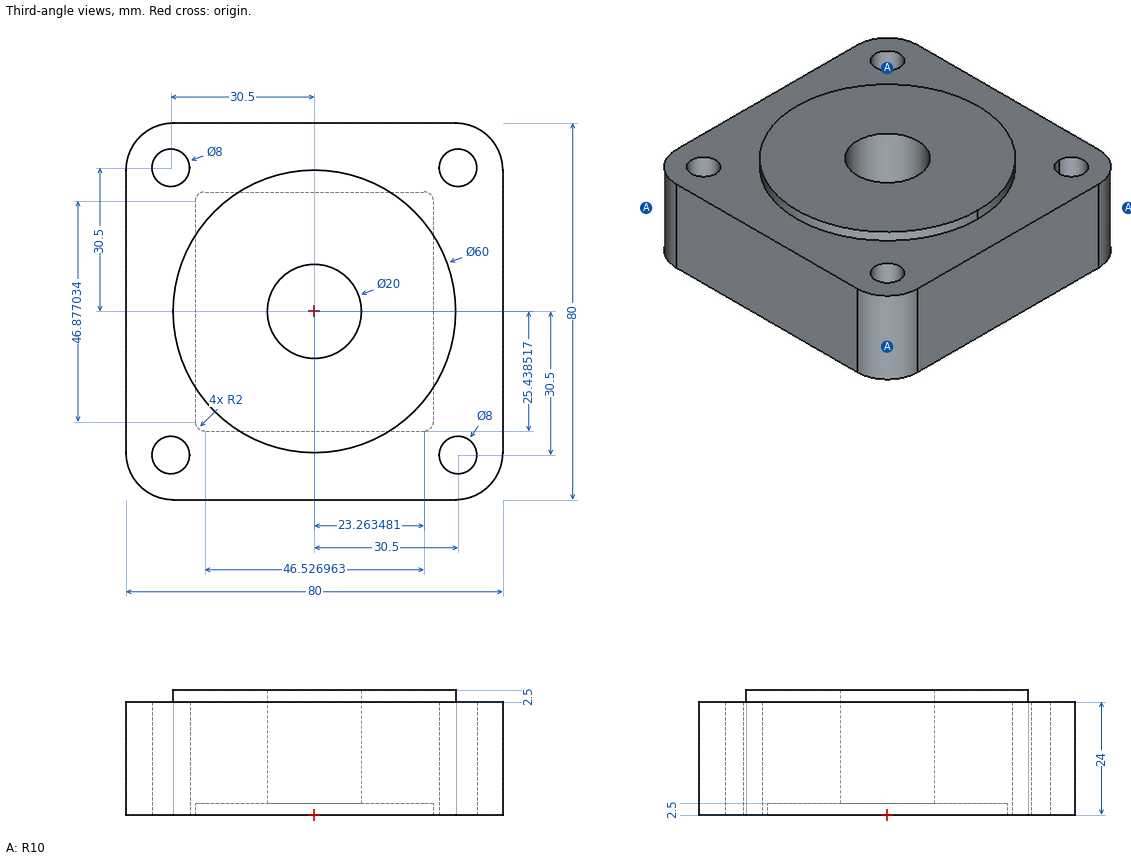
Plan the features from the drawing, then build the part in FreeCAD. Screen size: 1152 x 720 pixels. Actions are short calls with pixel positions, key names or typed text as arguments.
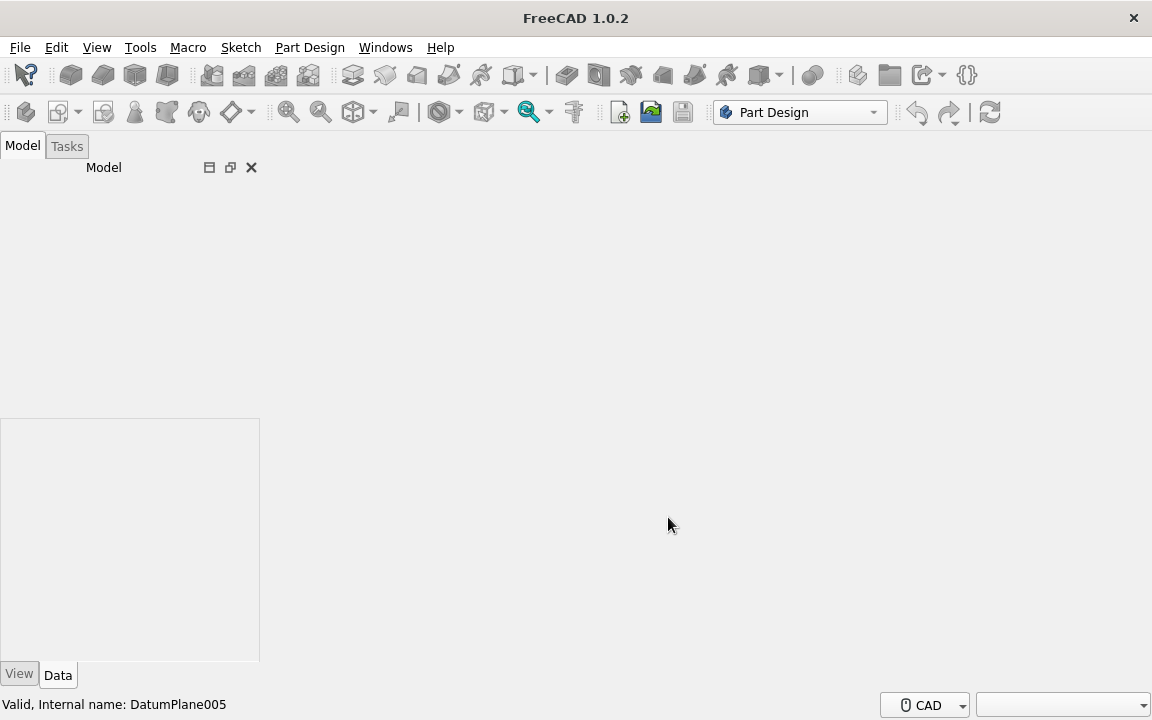
click(620, 112)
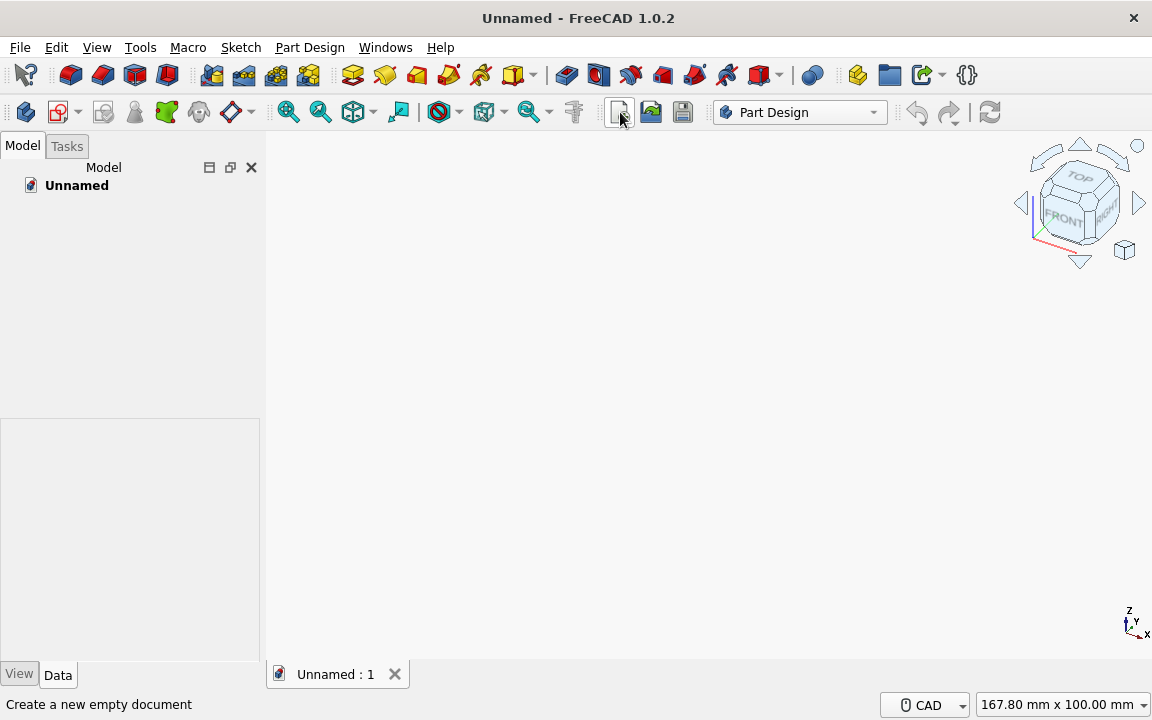
click(58, 112)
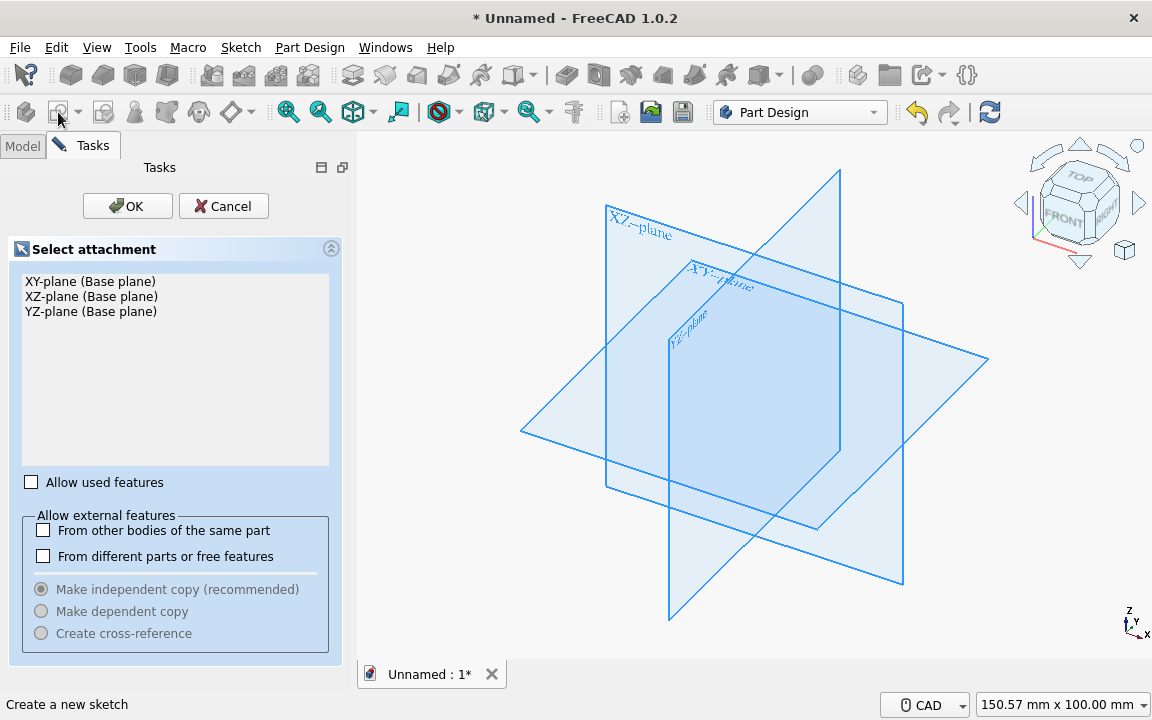
click(82, 282)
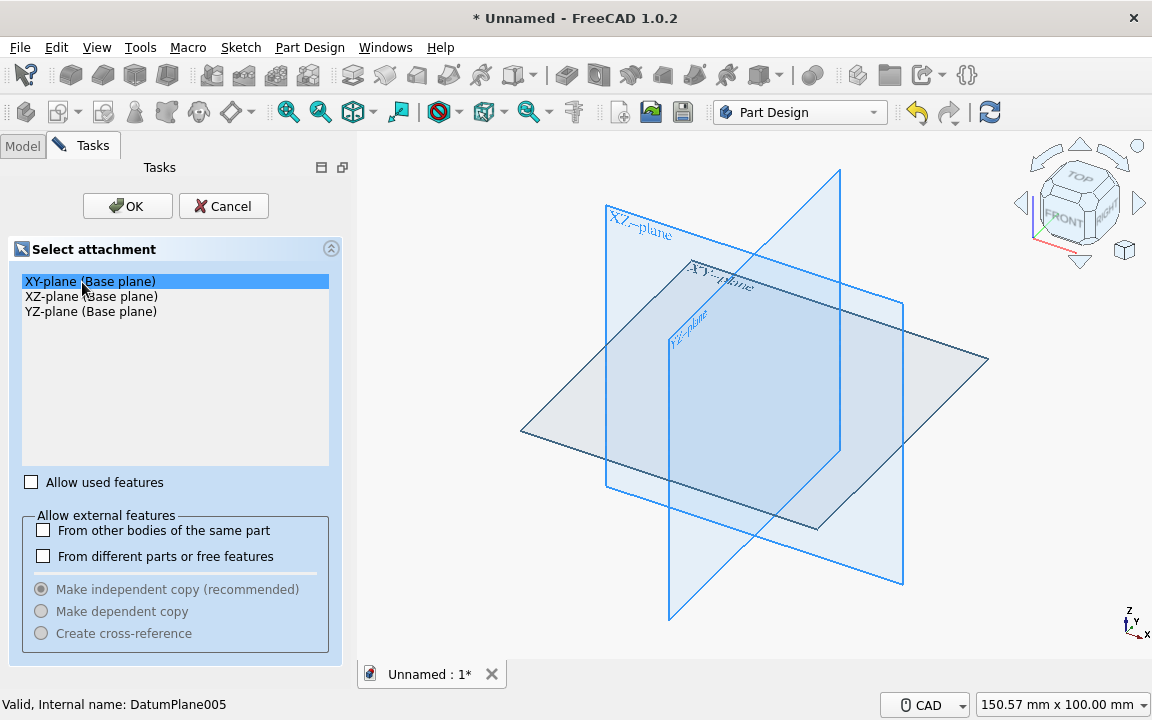
click(128, 206)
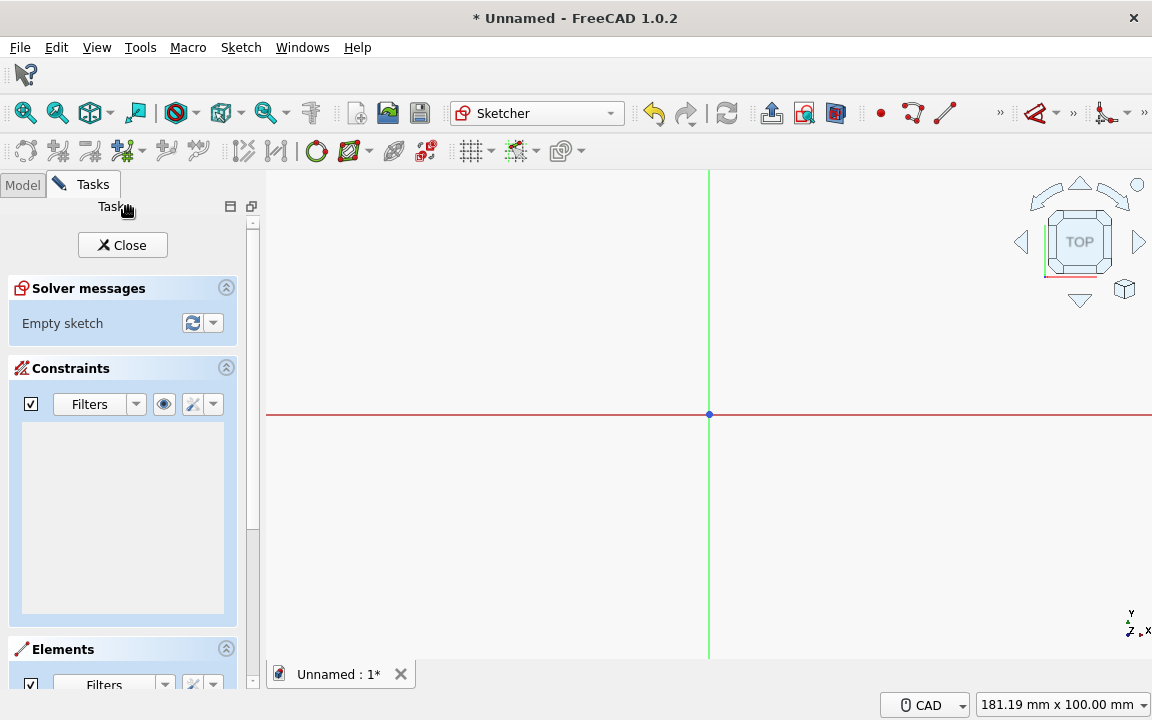
scroll(331, 415, down, 1)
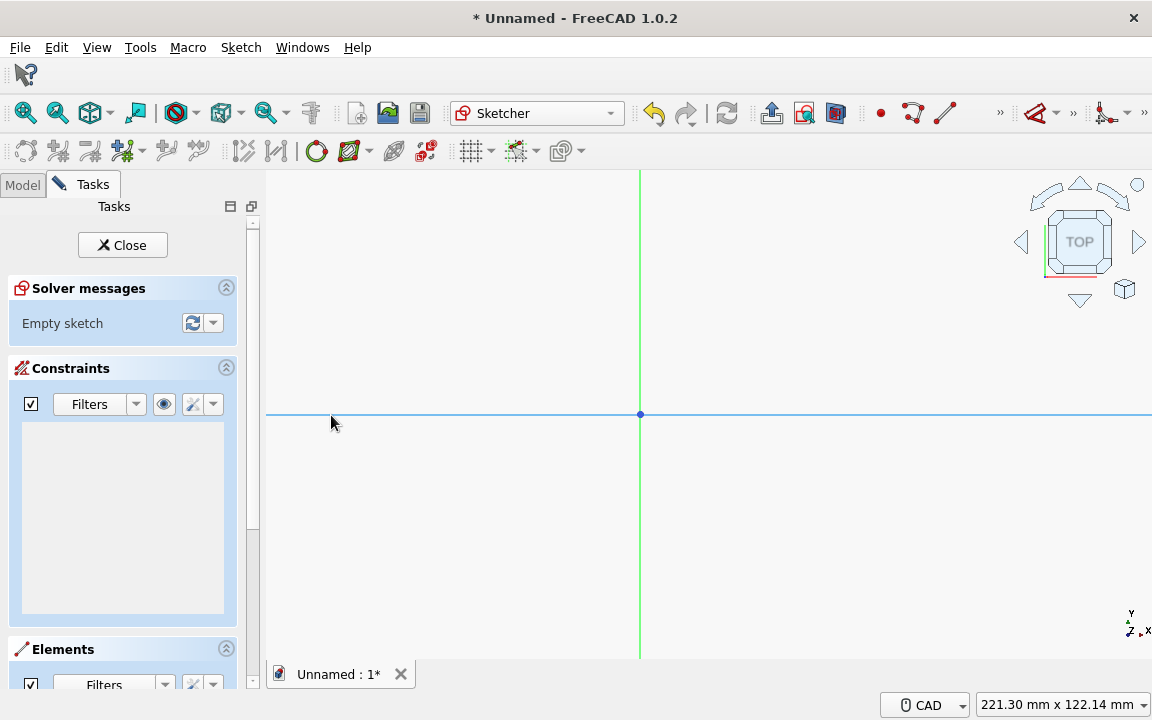
key(g)
key(v)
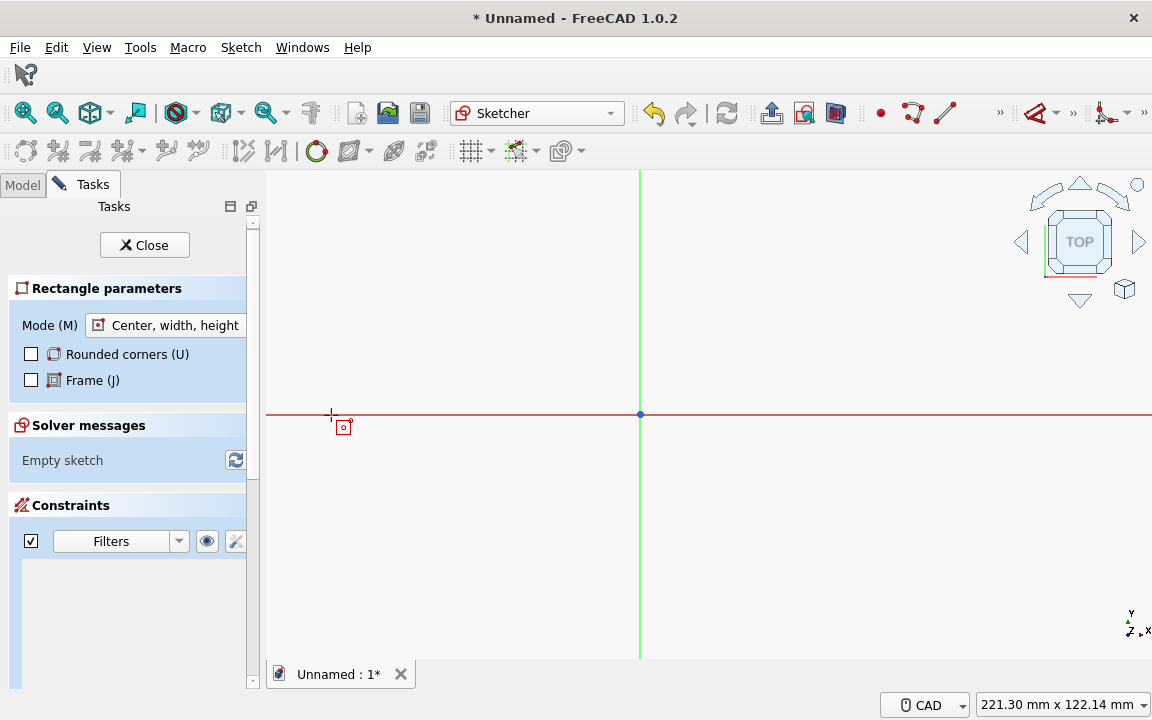
click(640, 415)
click(801, 255)
key(Escape)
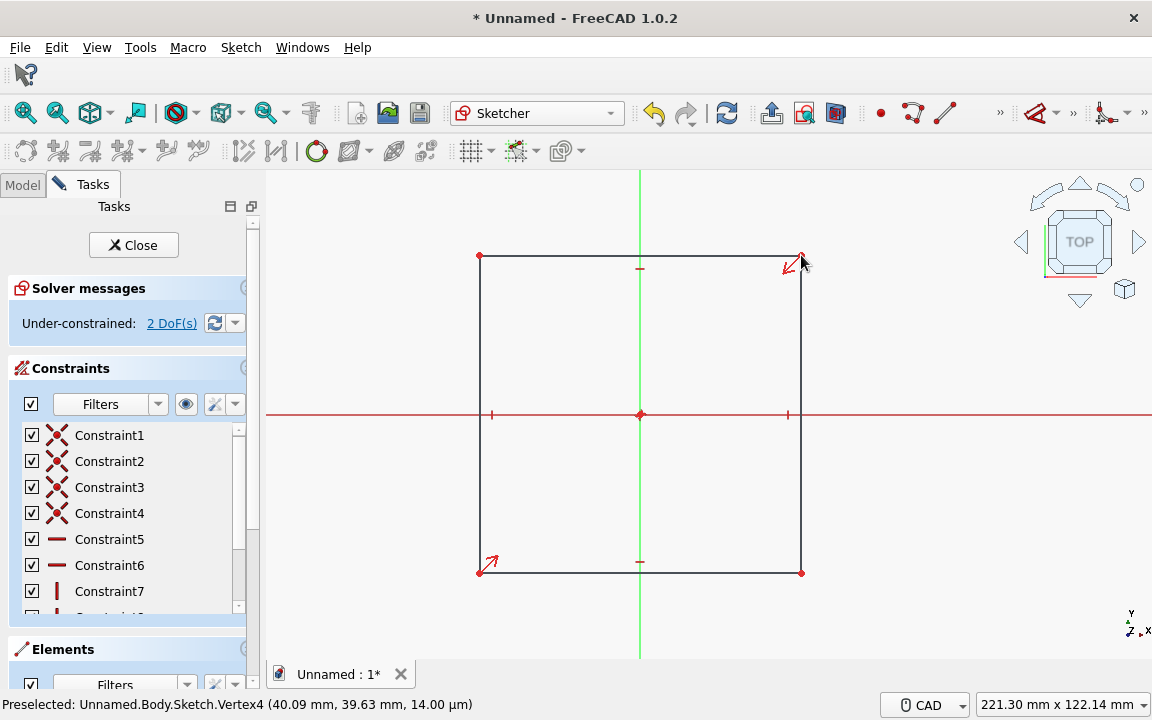
click(1036, 114)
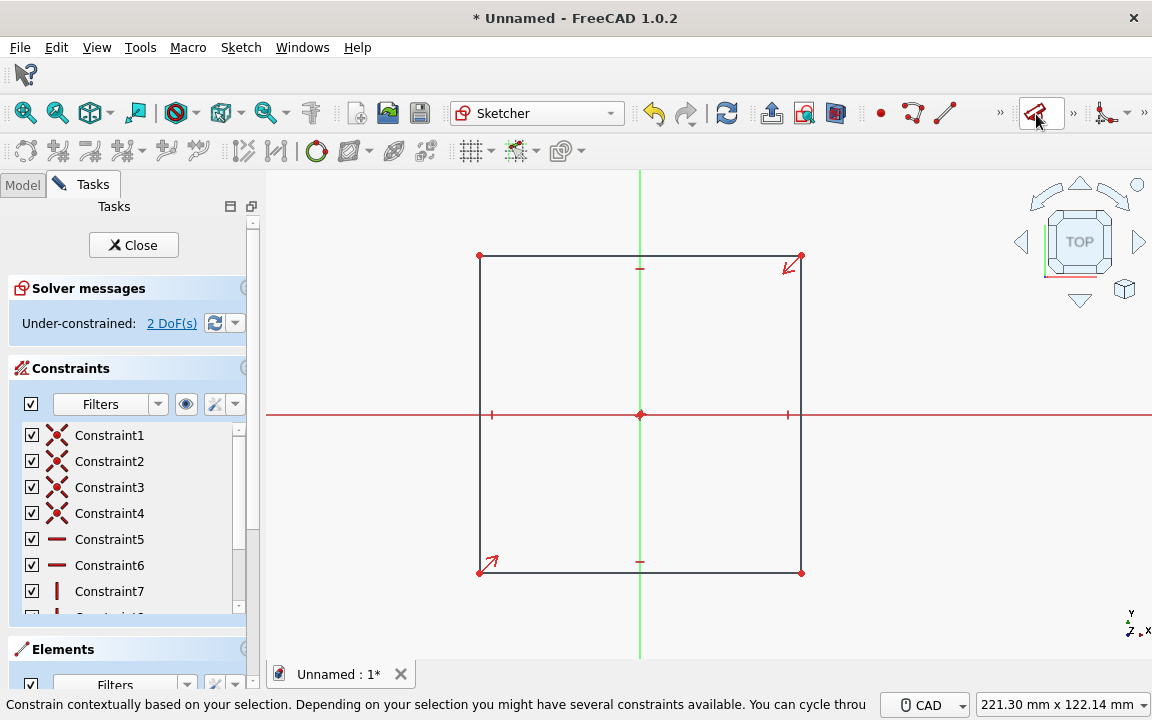
click(576, 573)
click(567, 607)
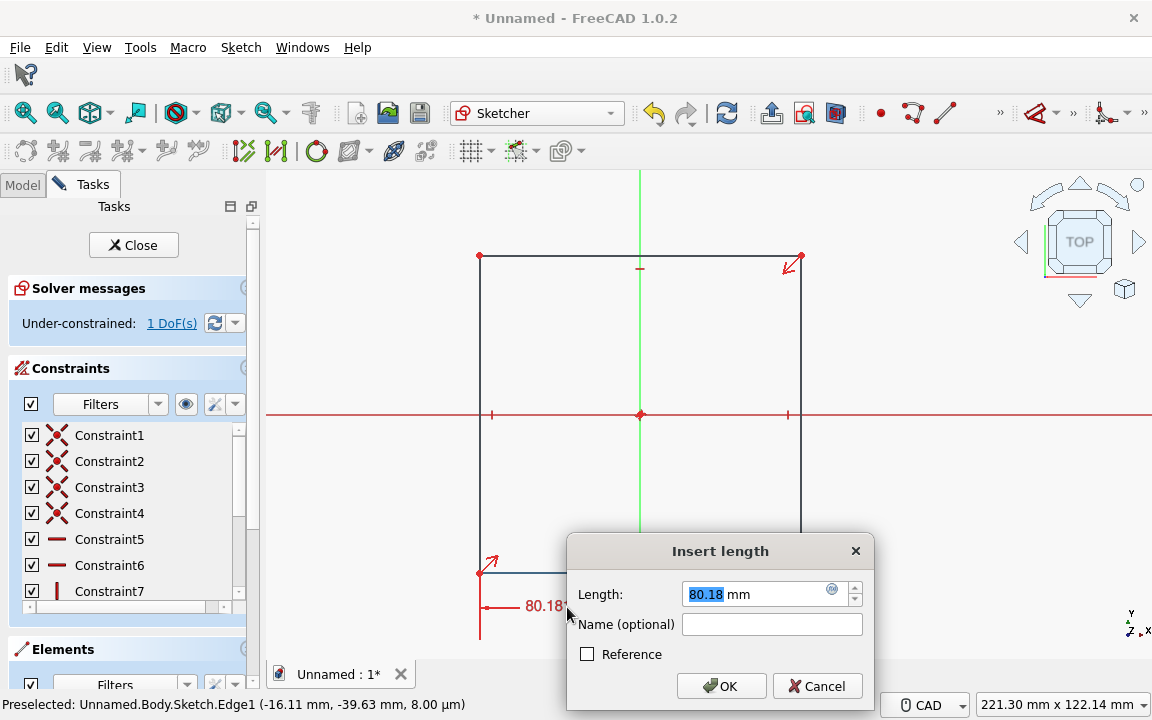
text(80)
key(Return)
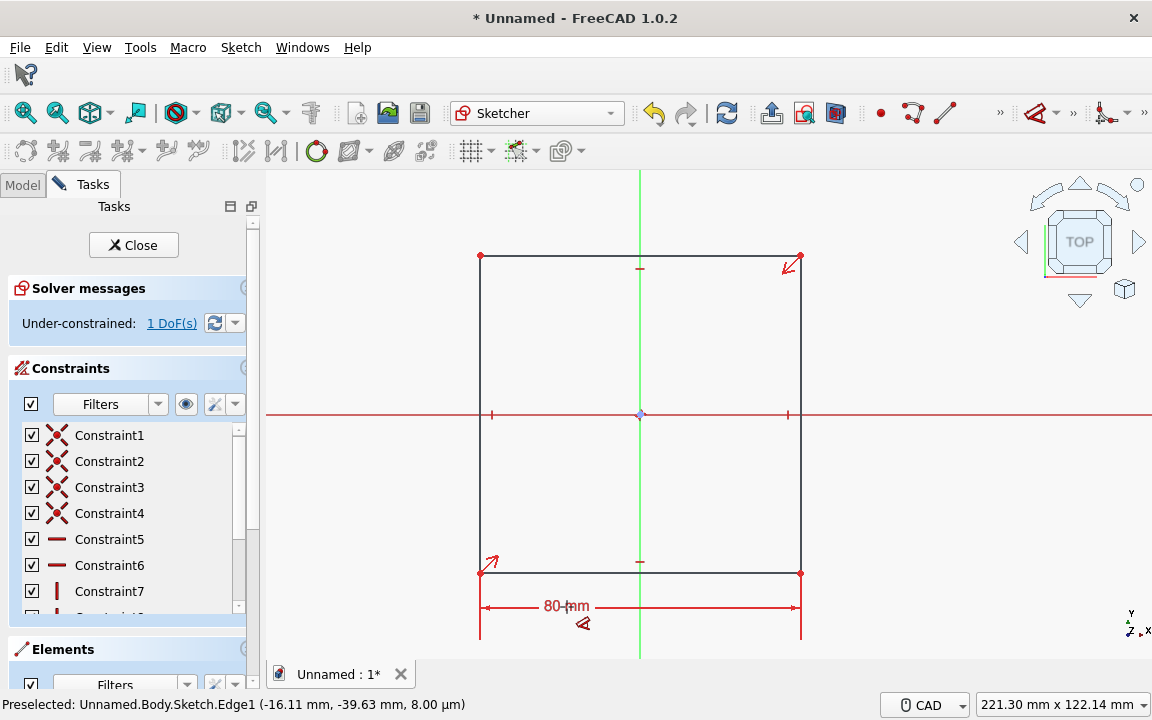
click(801, 478)
click(835, 342)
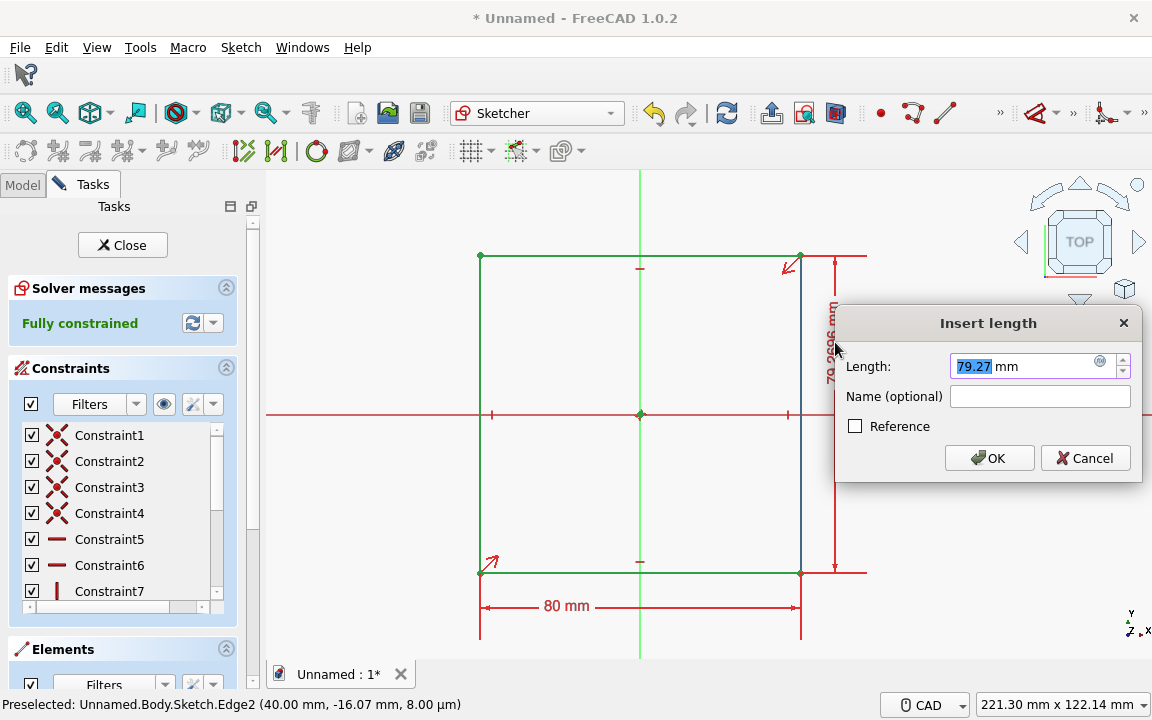
text(80)
key(Return)
key(Escape)